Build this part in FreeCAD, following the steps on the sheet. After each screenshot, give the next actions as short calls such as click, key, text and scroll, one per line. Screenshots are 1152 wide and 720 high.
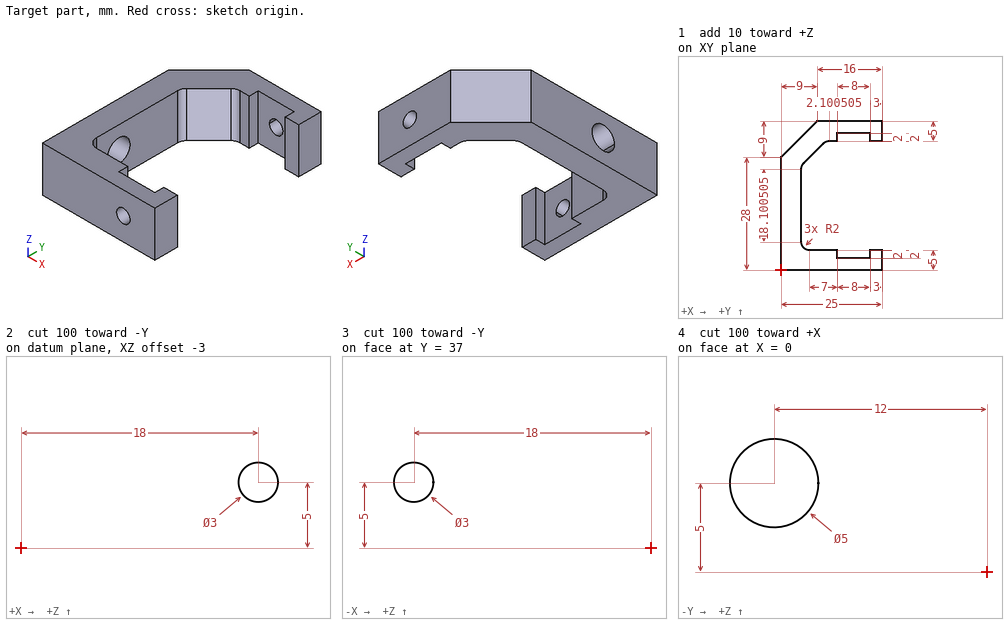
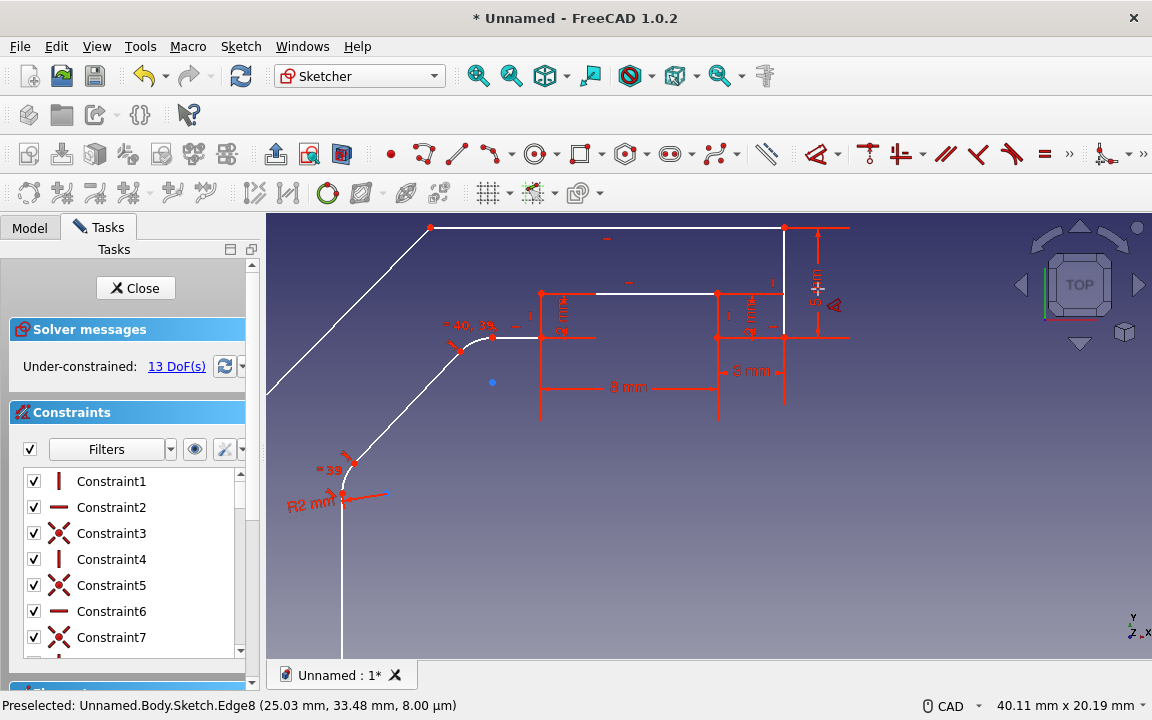
scroll(718, 318, down, 5)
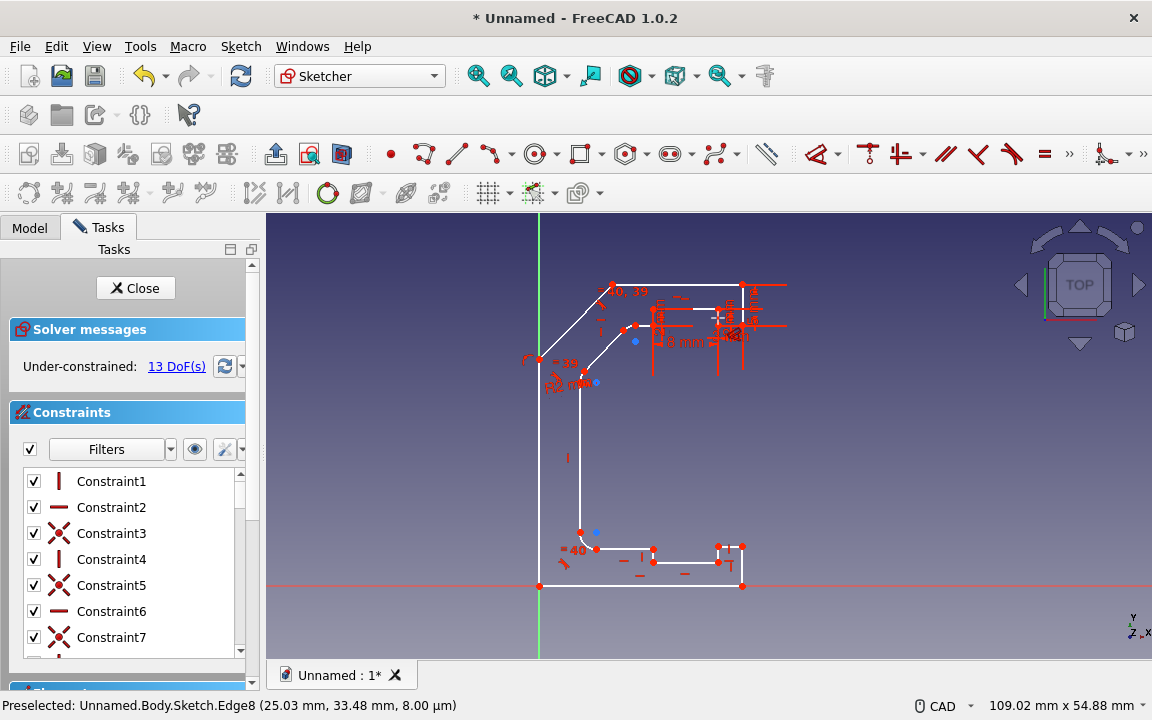
click(742, 574)
click(776, 567)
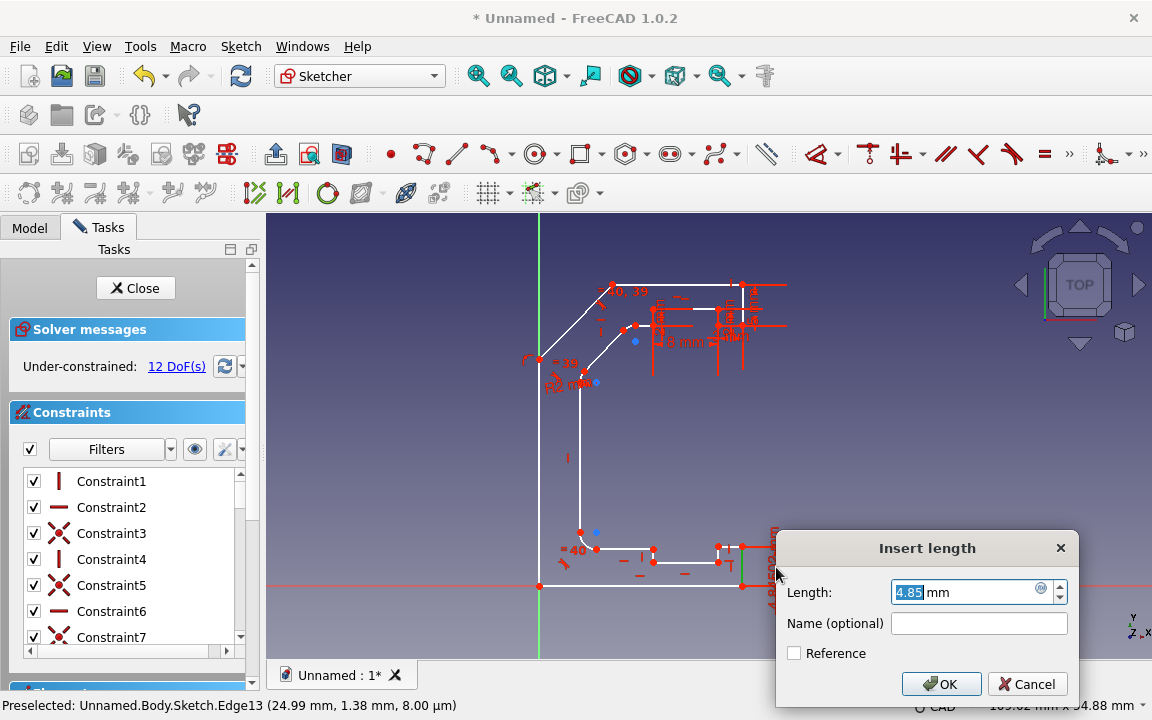
text(5)
key(Return)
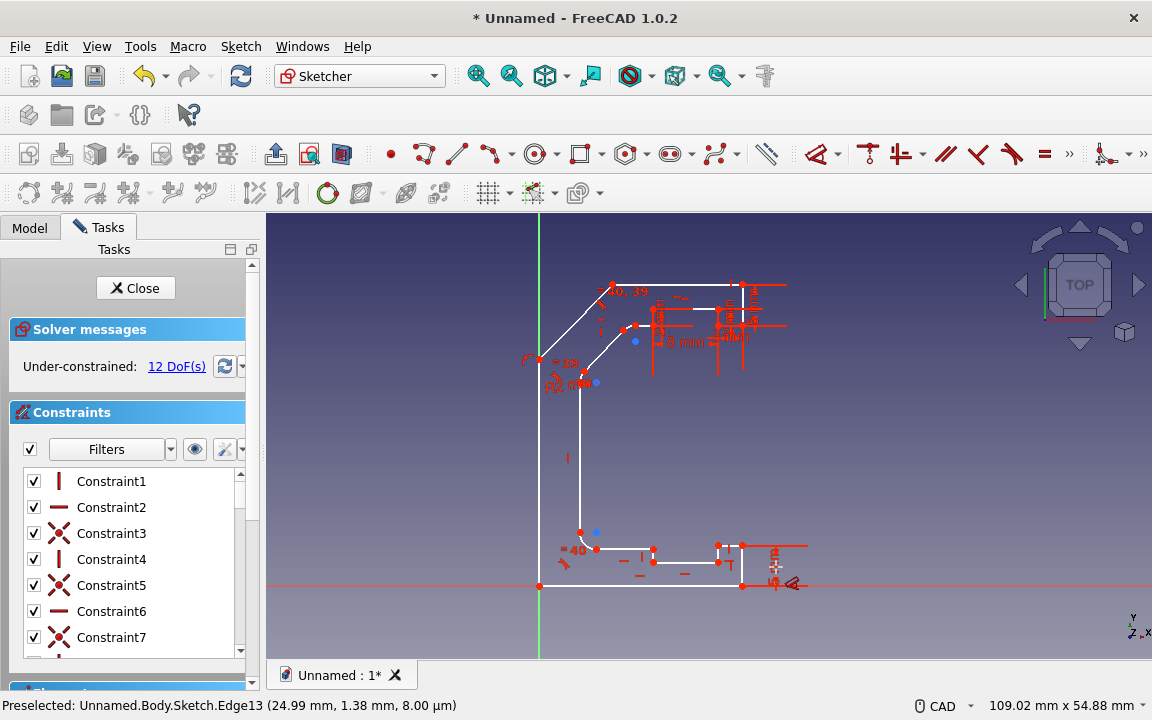
scroll(733, 546, up, 3)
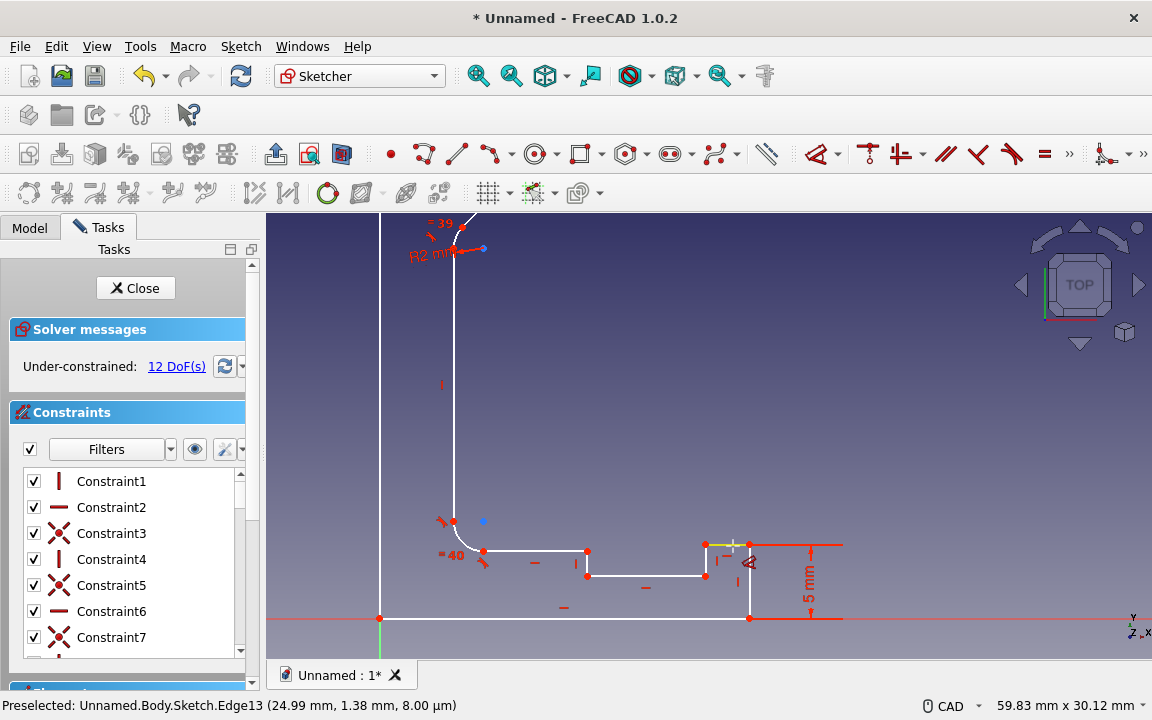
click(732, 545)
click(728, 579)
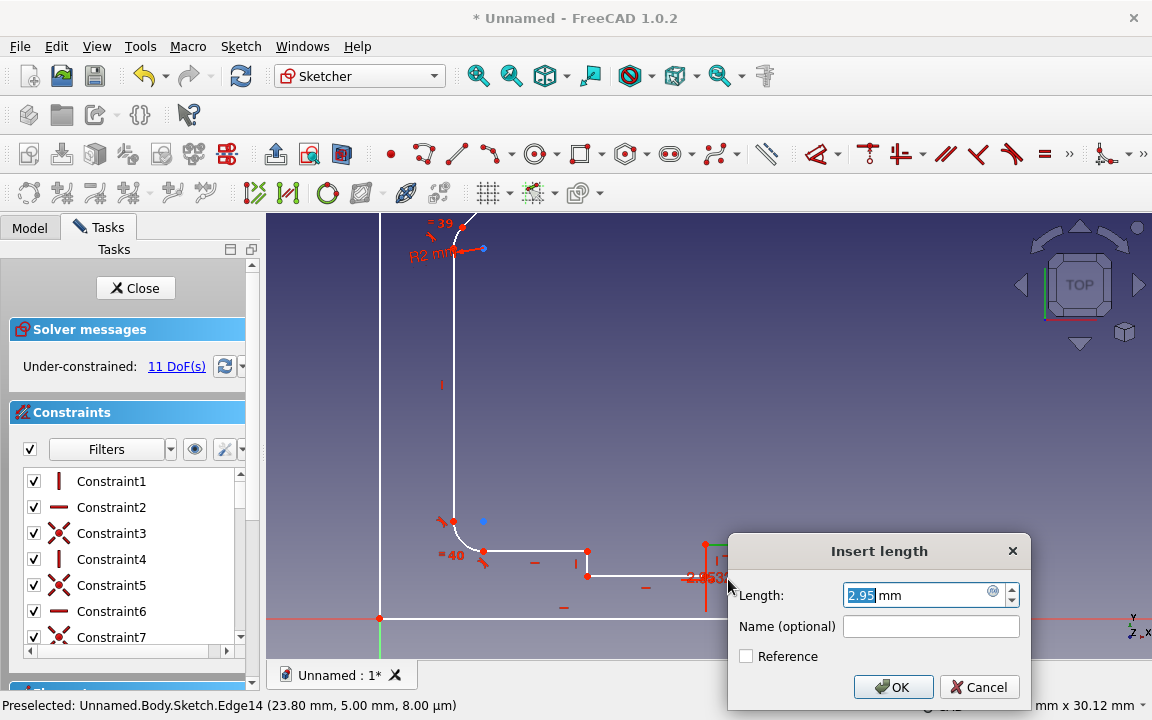
text(3)
key(Return)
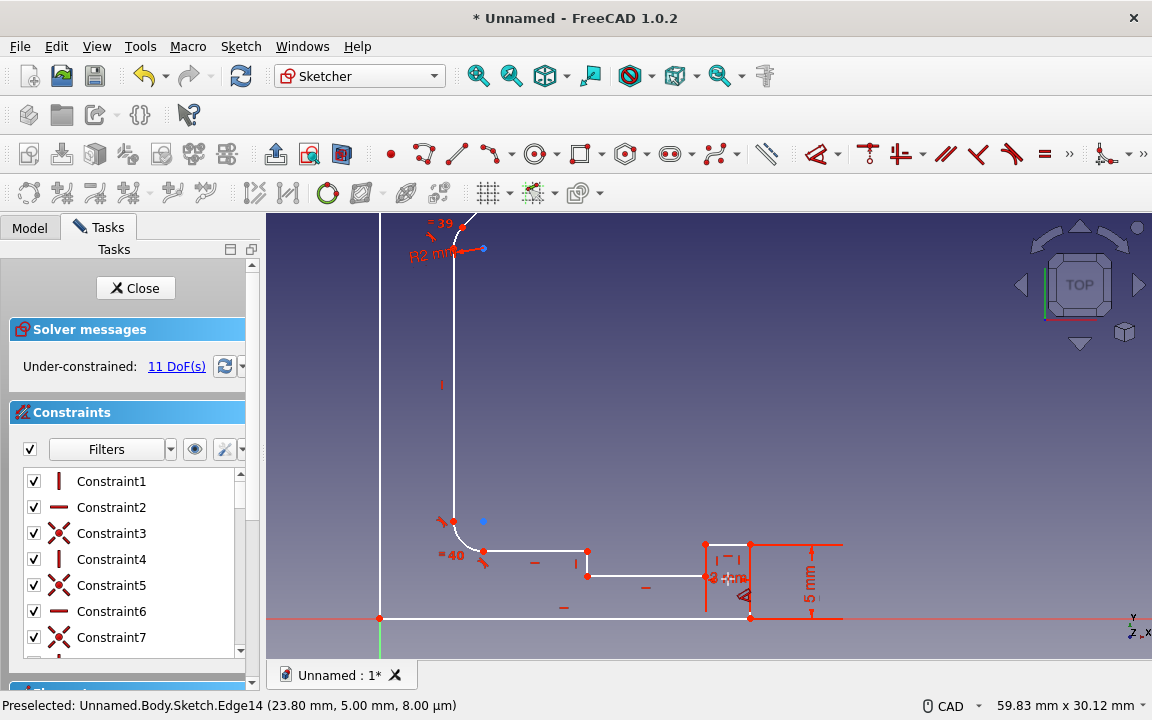
scroll(706, 554, up, 2)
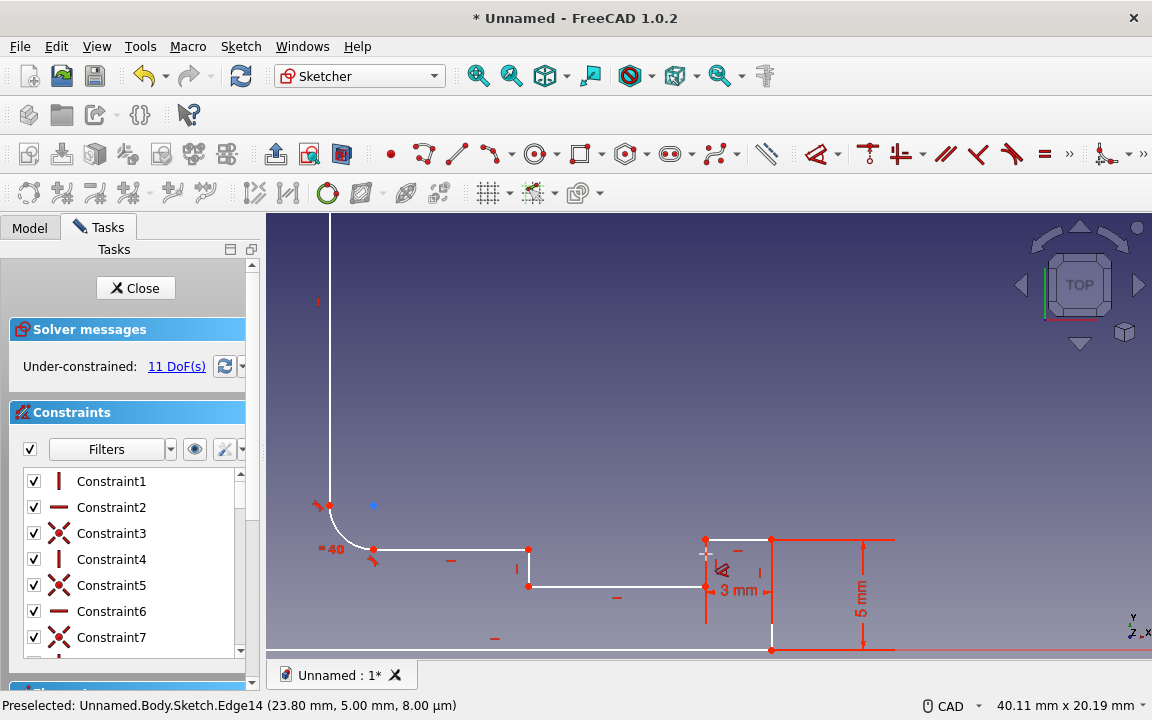
click(706, 554)
click(740, 563)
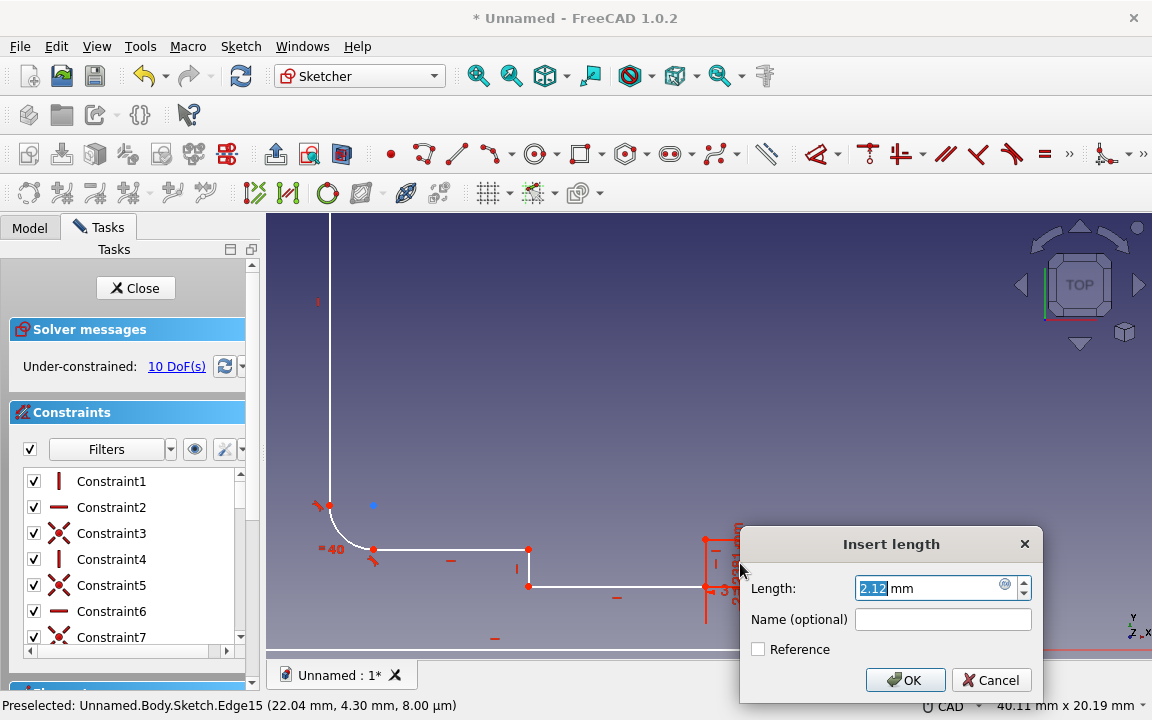
text(2)
key(Return)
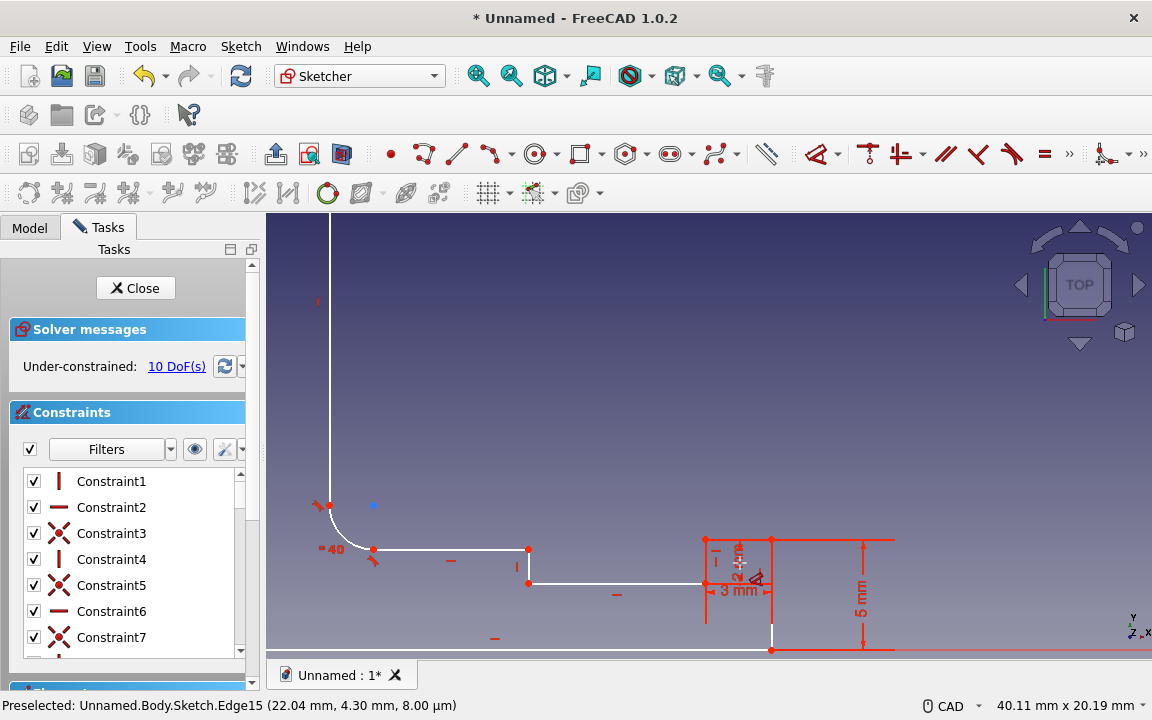
click(653, 584)
click(617, 618)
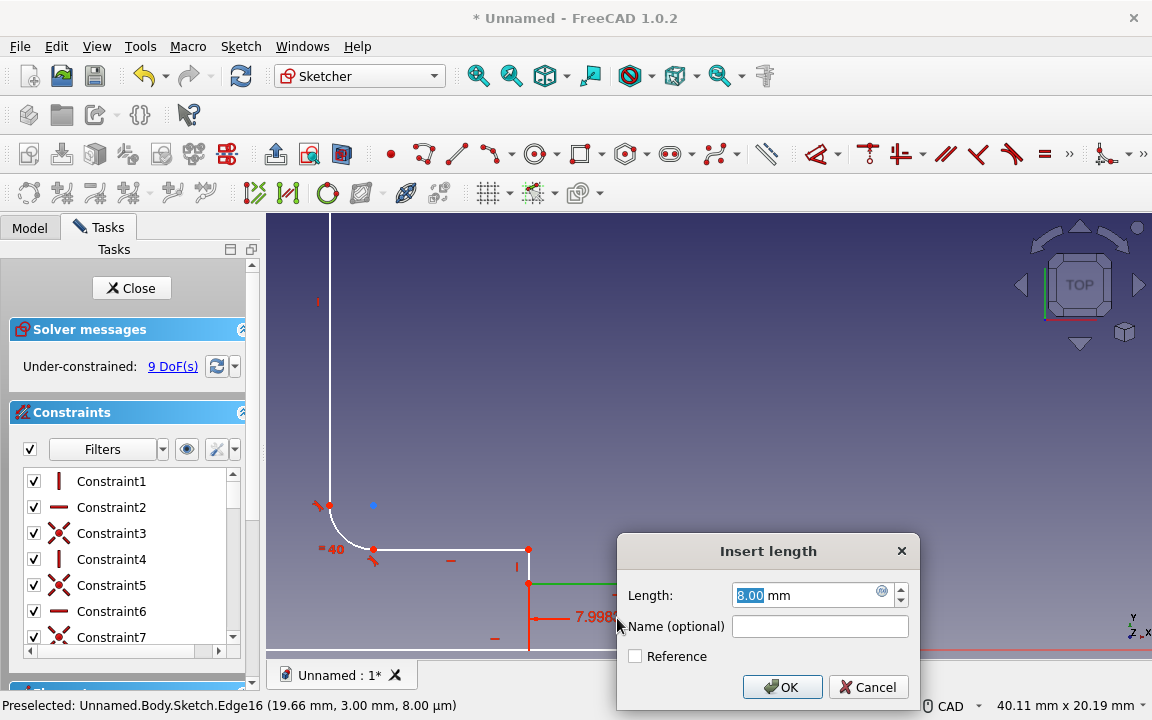
text(8)
key(Return)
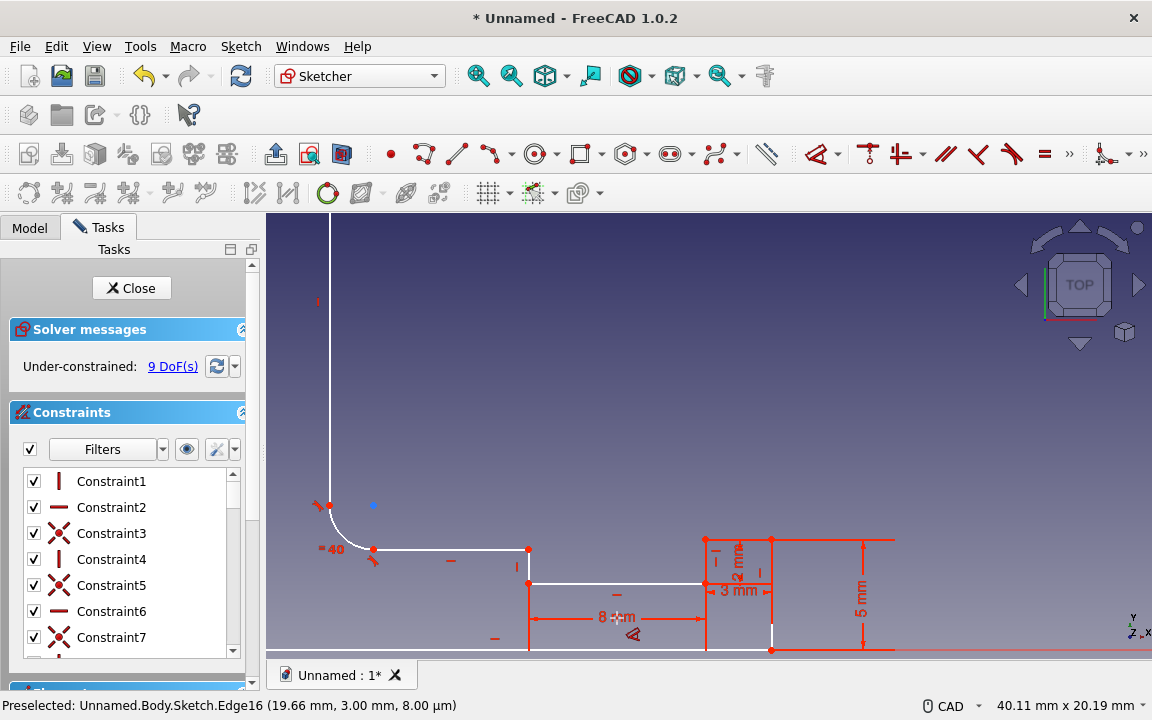
scroll(529, 574, up, 2)